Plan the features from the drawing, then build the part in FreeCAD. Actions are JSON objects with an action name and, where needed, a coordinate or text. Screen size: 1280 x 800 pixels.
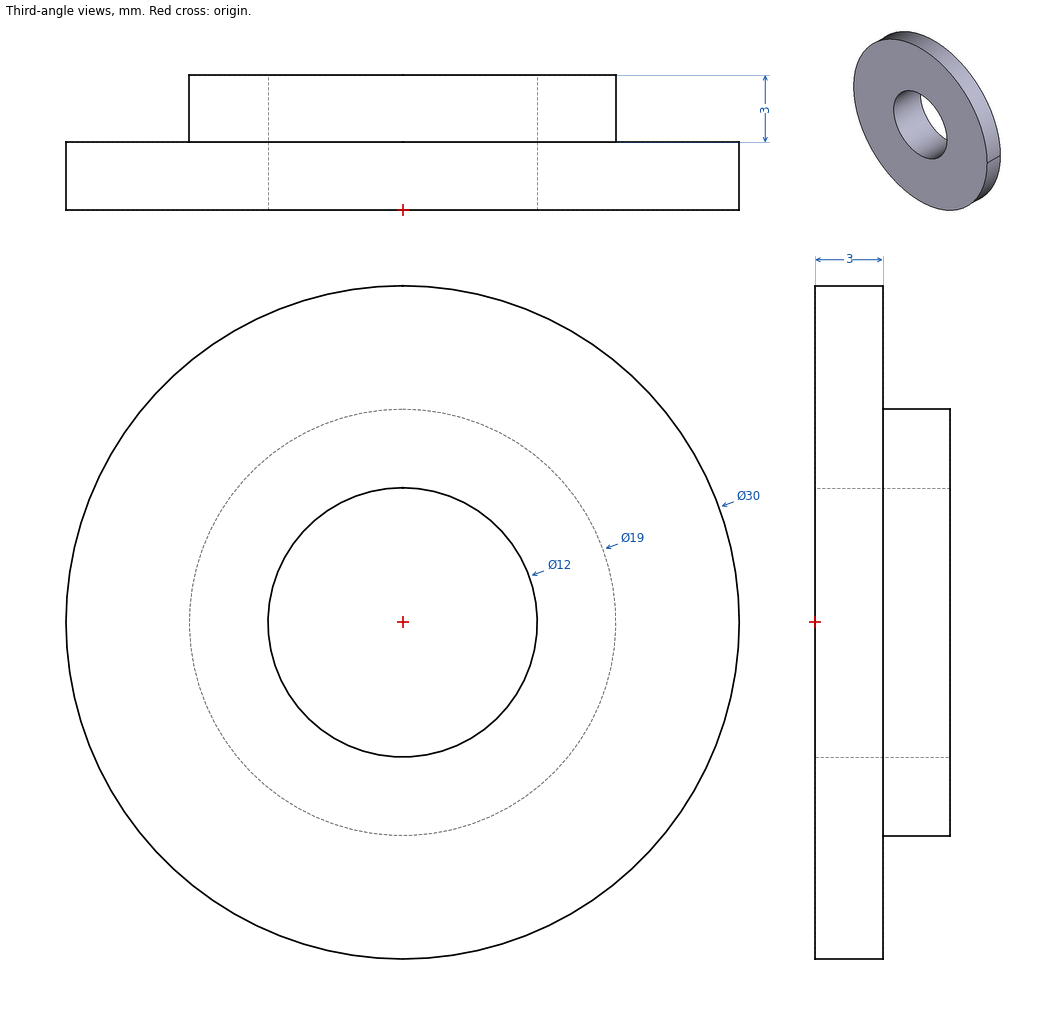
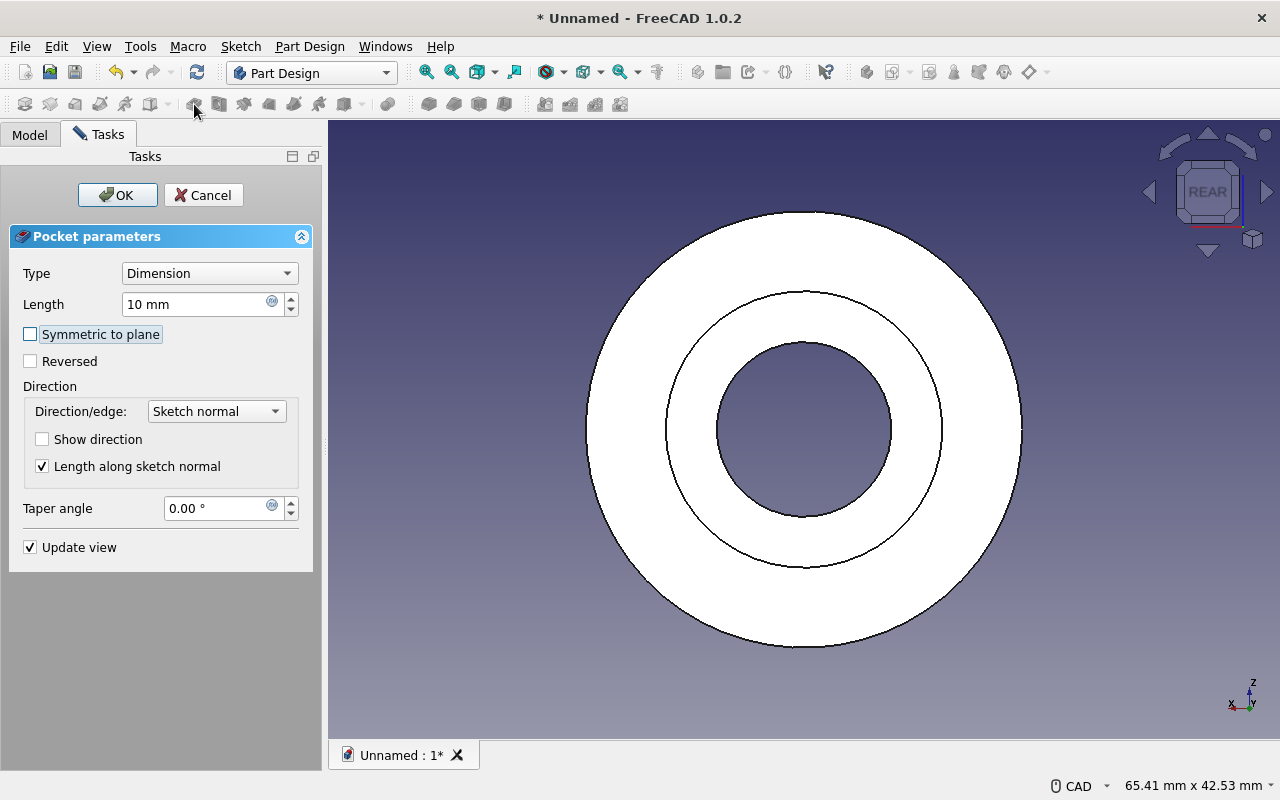
{"action": "left_click", "coordinate": [118, 195]}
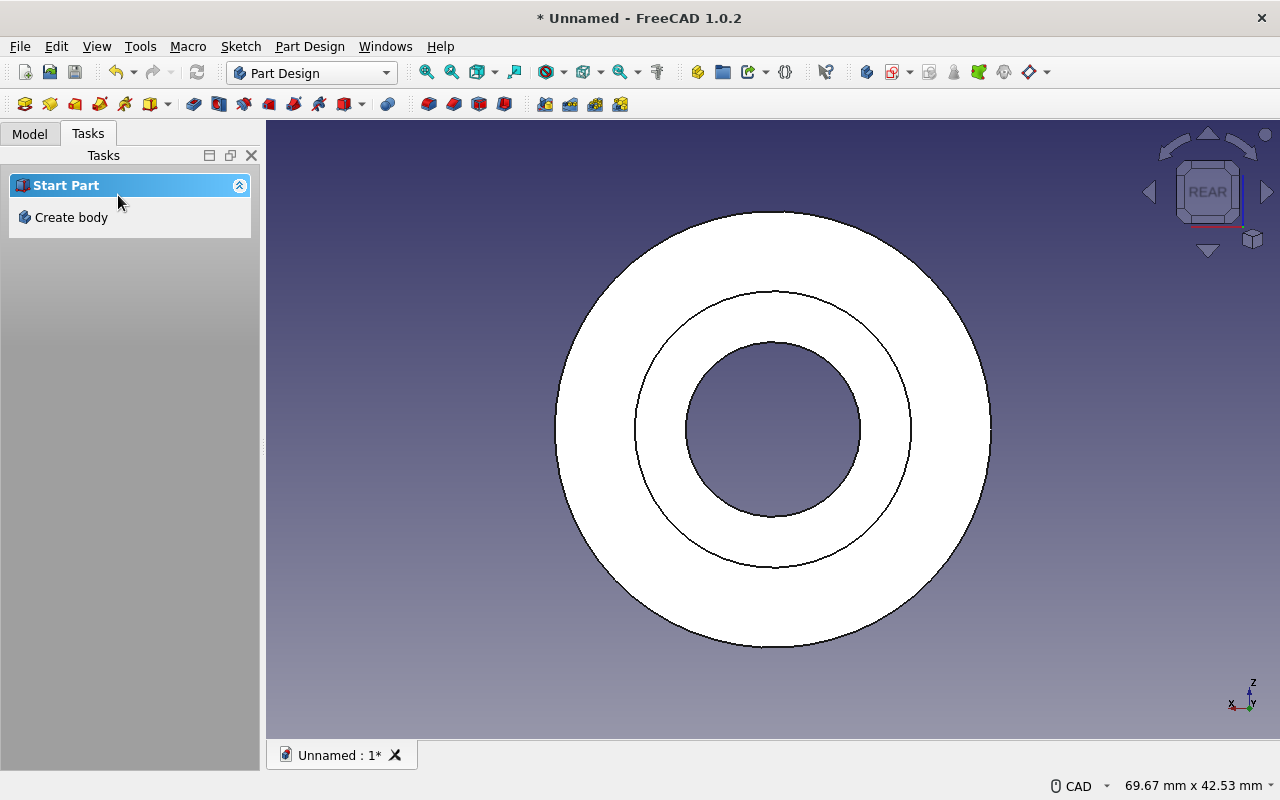
{"action": "key", "text": "0"}